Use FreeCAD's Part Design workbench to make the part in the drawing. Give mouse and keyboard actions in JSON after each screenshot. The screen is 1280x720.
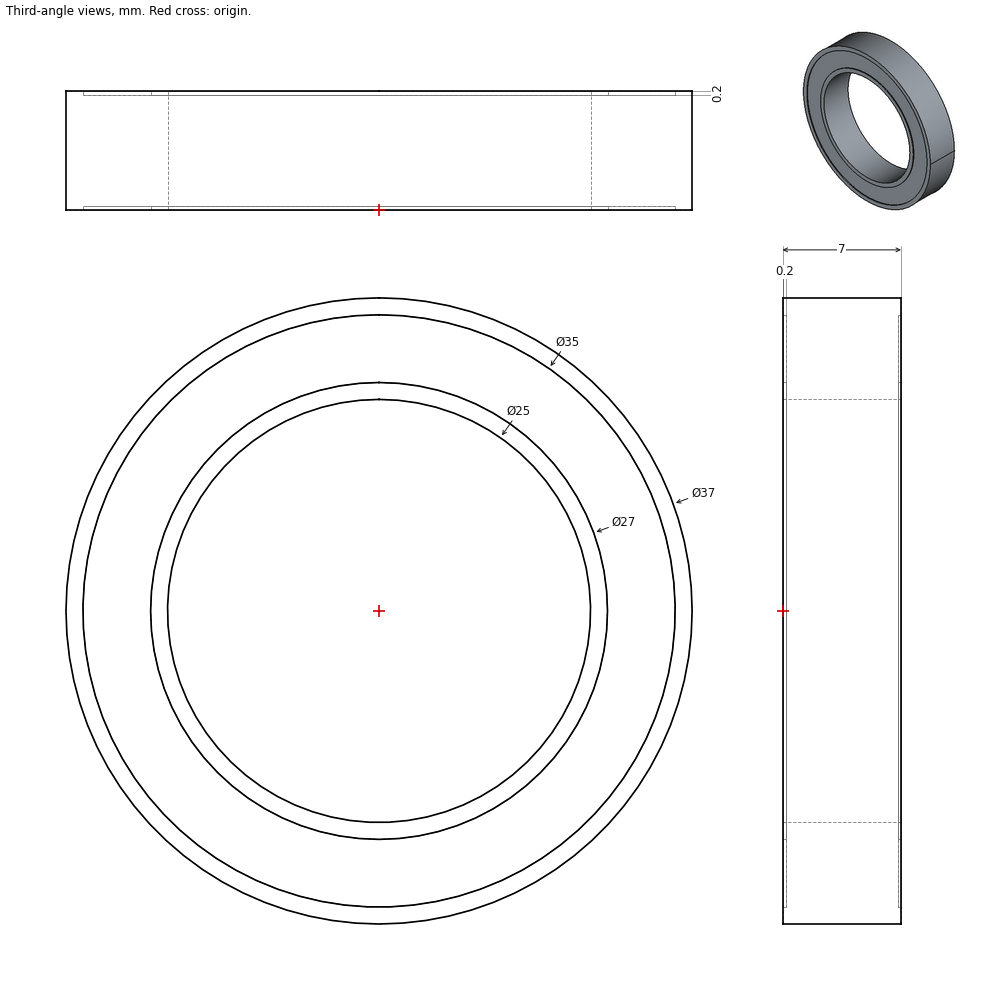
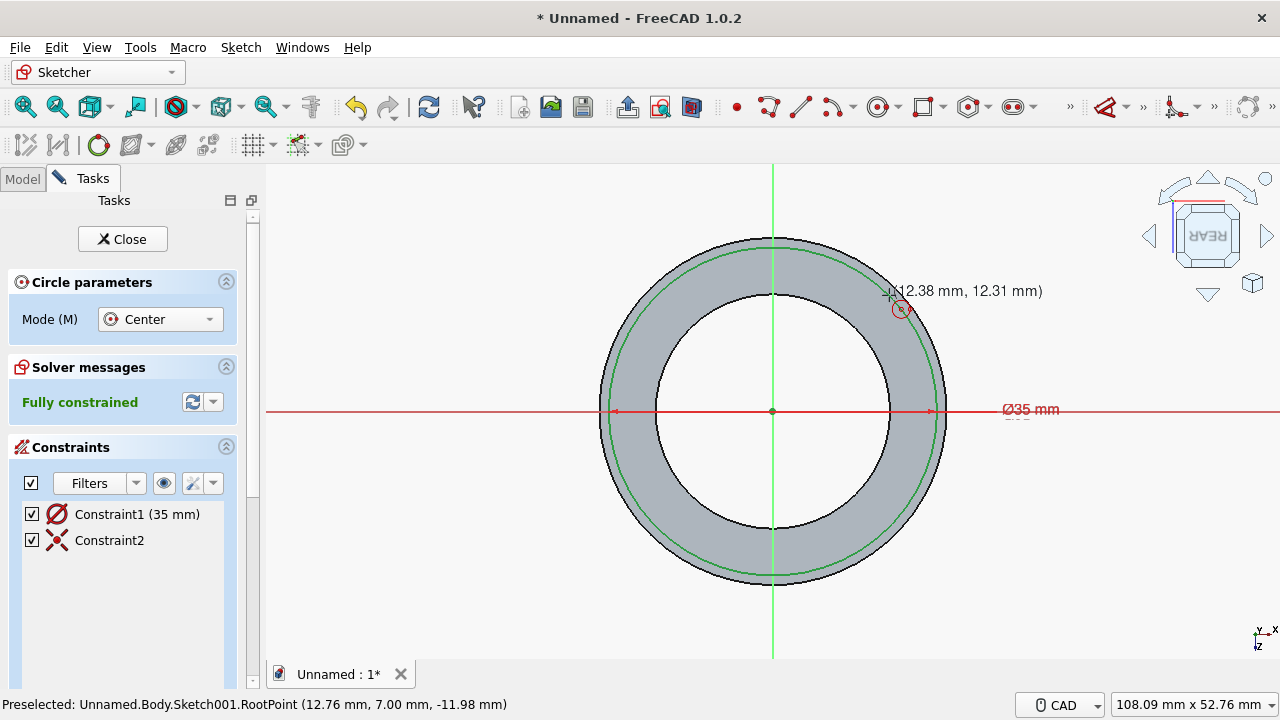
{"action": "left_click", "coordinate": [773, 411]}
{"action": "mouse_move", "coordinate": [862, 322]}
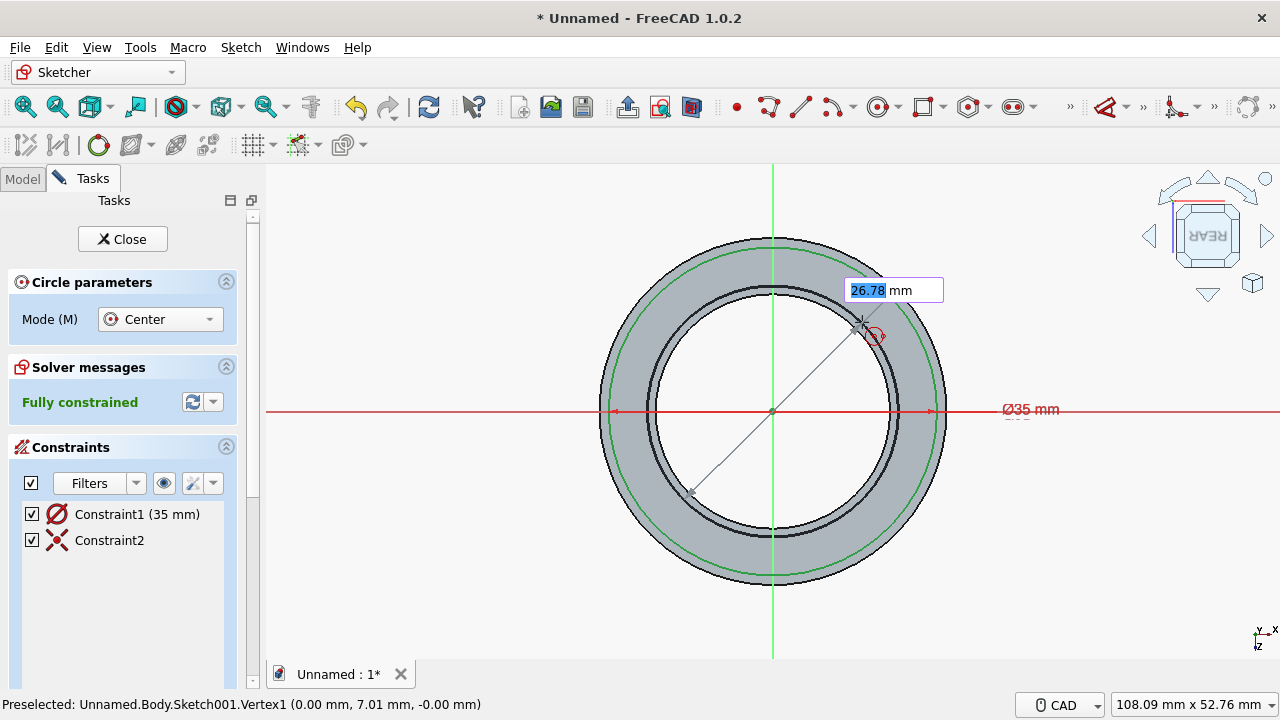
{"action": "type", "text": "27"}
{"action": "key", "text": "Return"}
{"action": "key", "text": "Escape"}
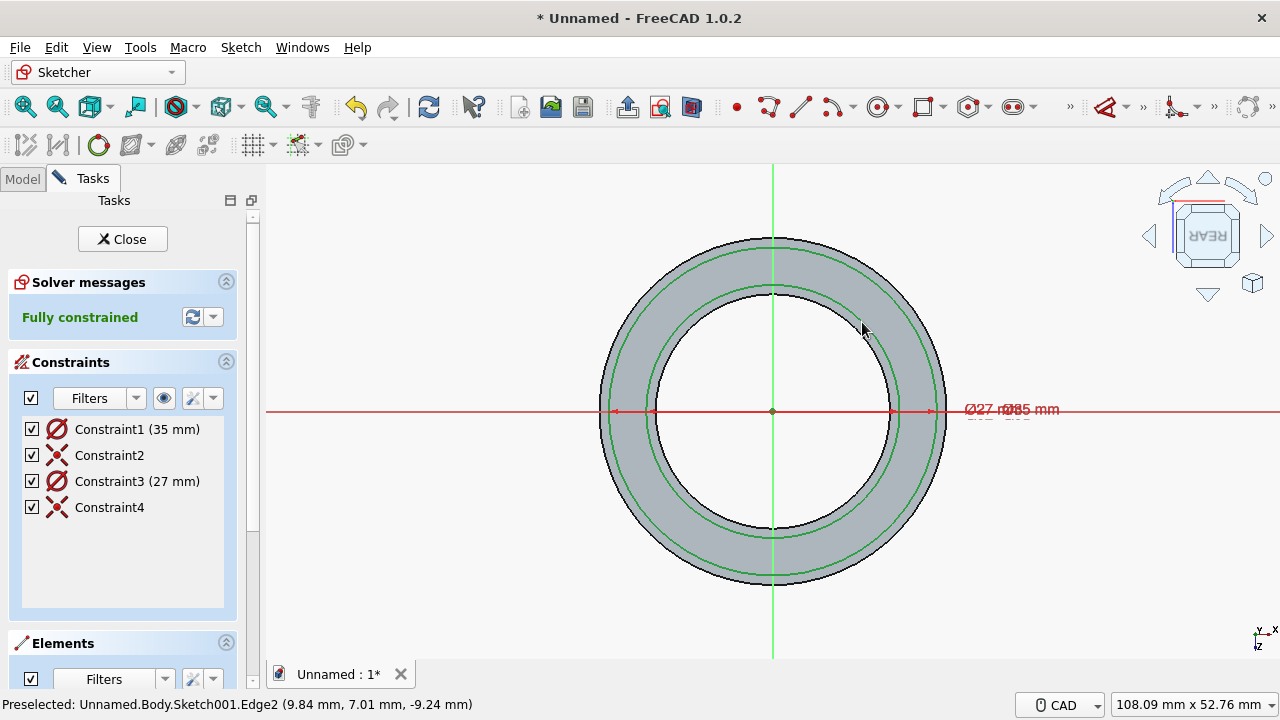
{"action": "left_click", "coordinate": [123, 239]}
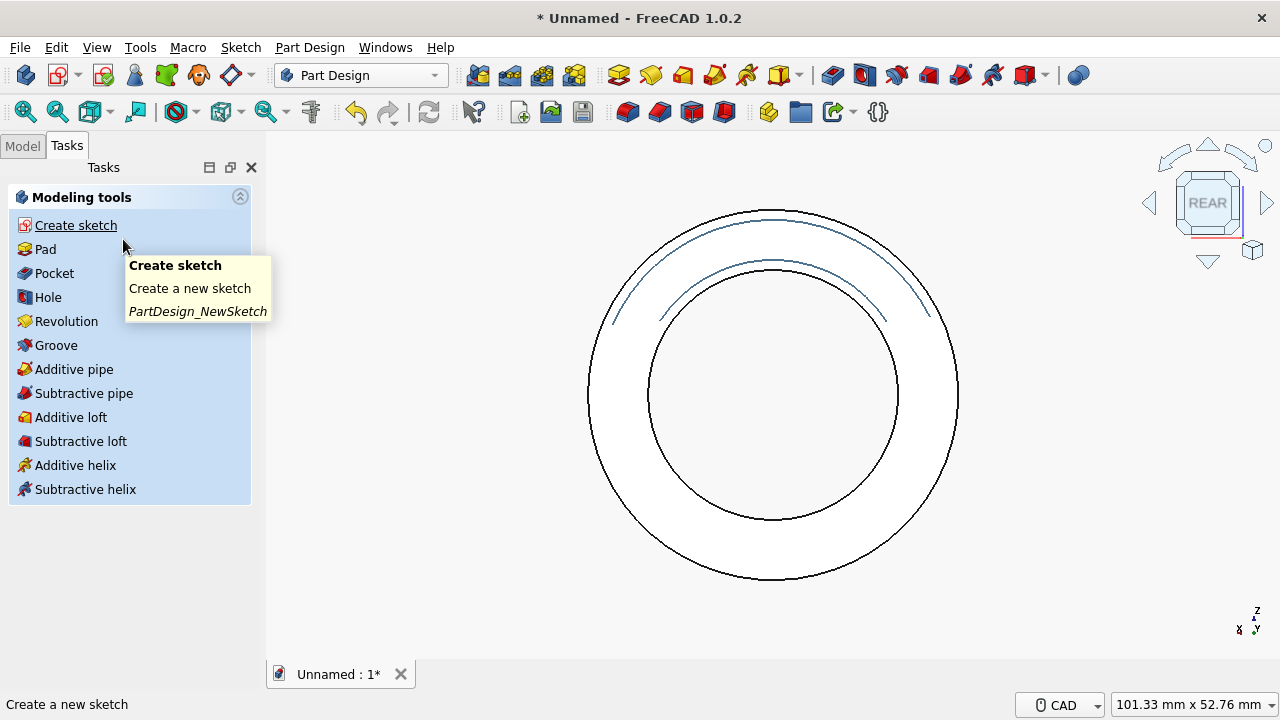
{"action": "left_click", "coordinate": [834, 76]}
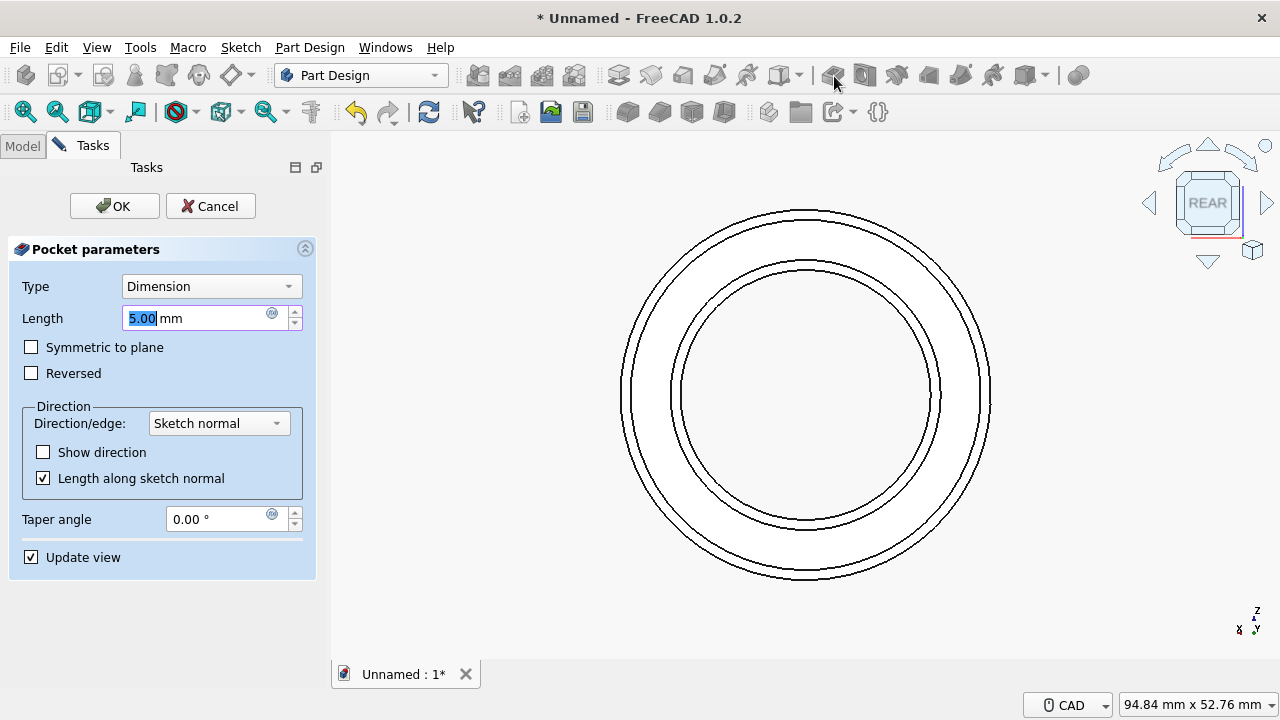
{"action": "type", "text": "0.2"}
{"action": "key", "text": "Tab"}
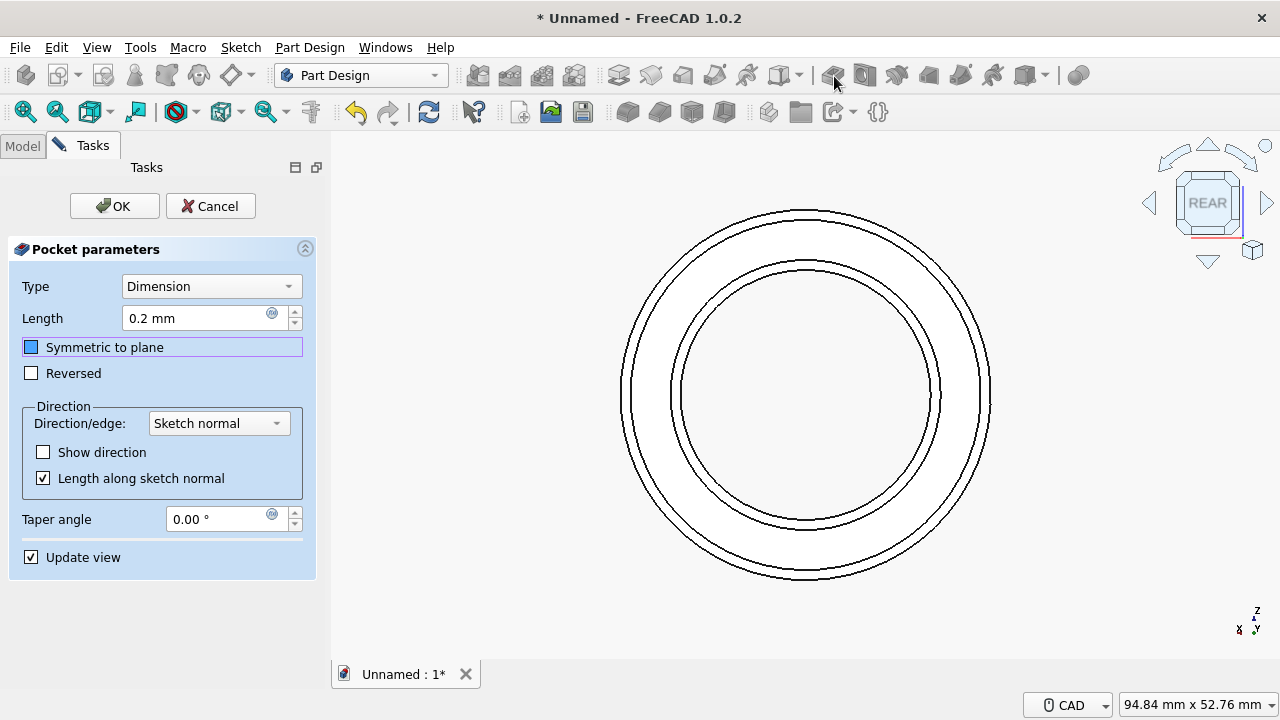
{"action": "left_click", "coordinate": [115, 206]}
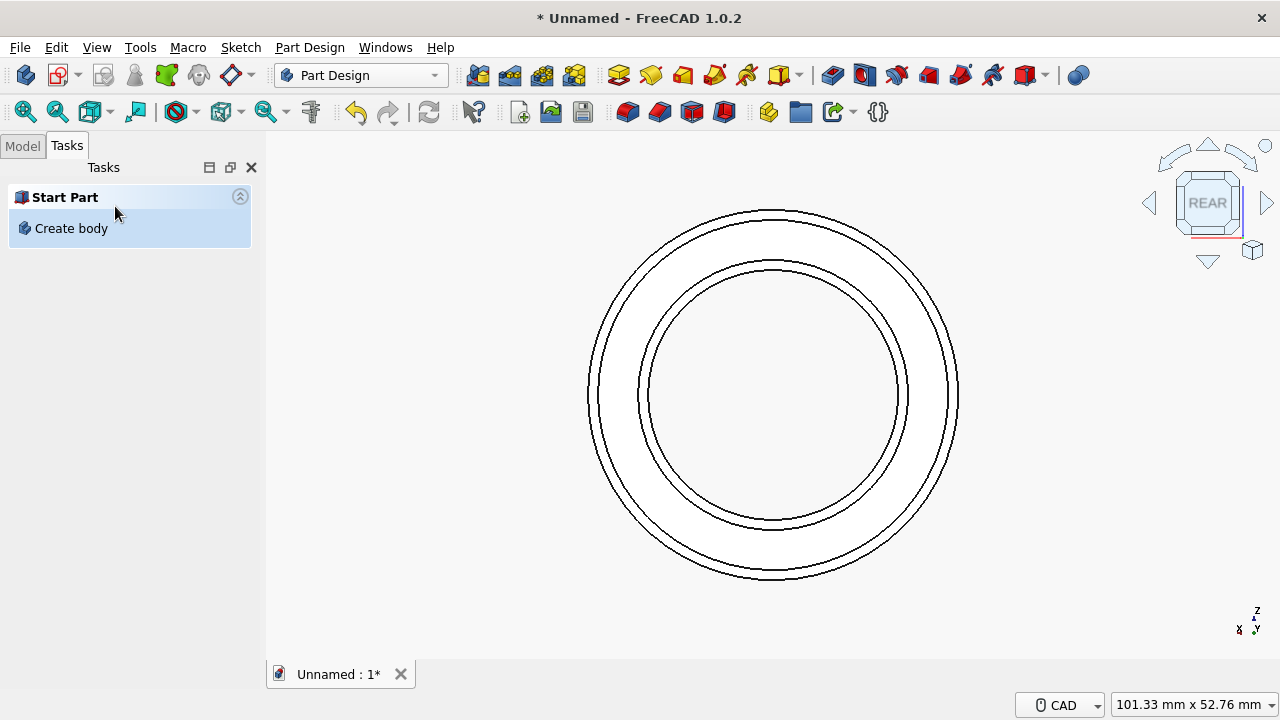
{"action": "left_click", "coordinate": [23, 145]}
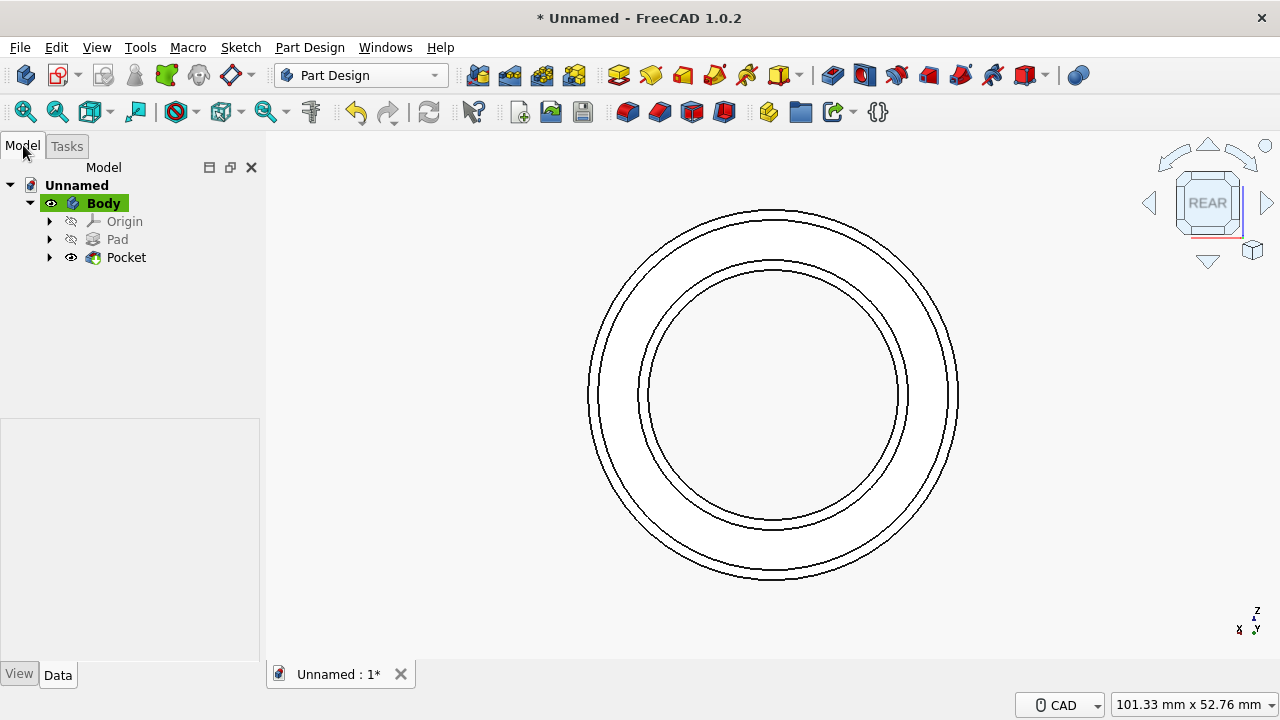
{"action": "left_click", "coordinate": [50, 221]}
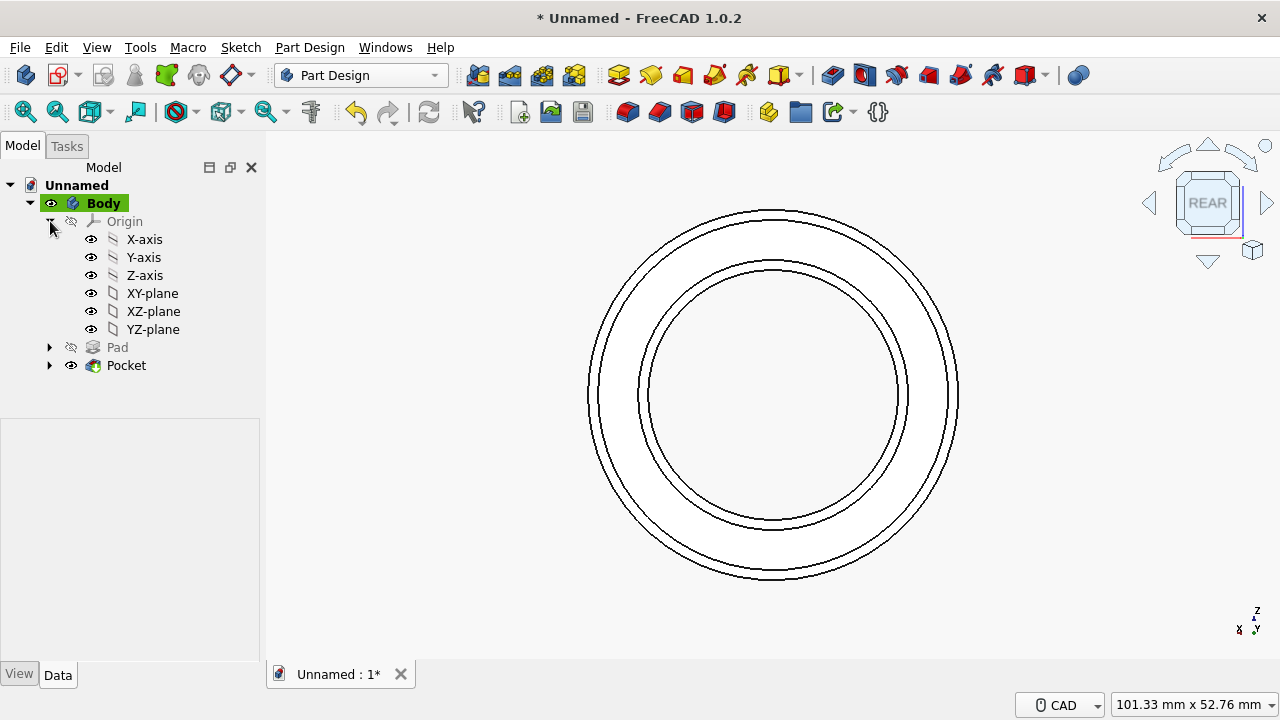
{"action": "left_click", "coordinate": [136, 311]}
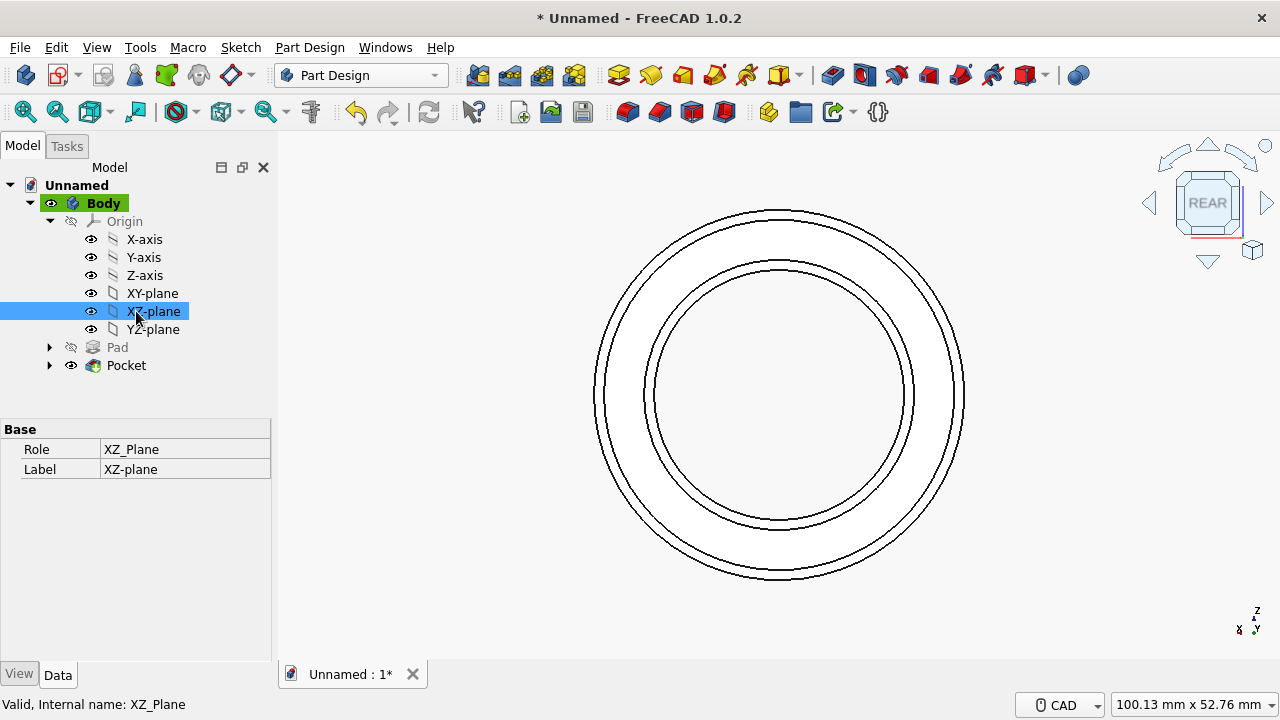
{"action": "left_click", "coordinate": [232, 76]}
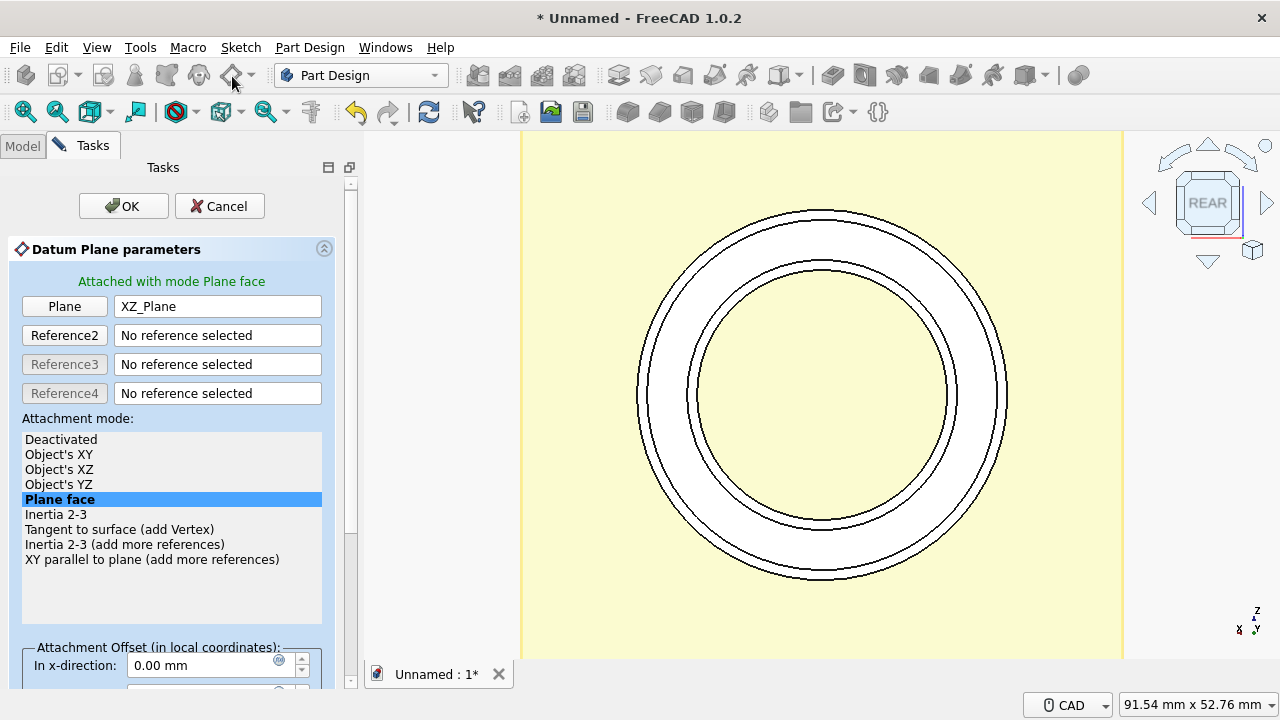
{"action": "scroll", "coordinate": [351, 432], "scroll_direction": "down", "scroll_amount": 2}